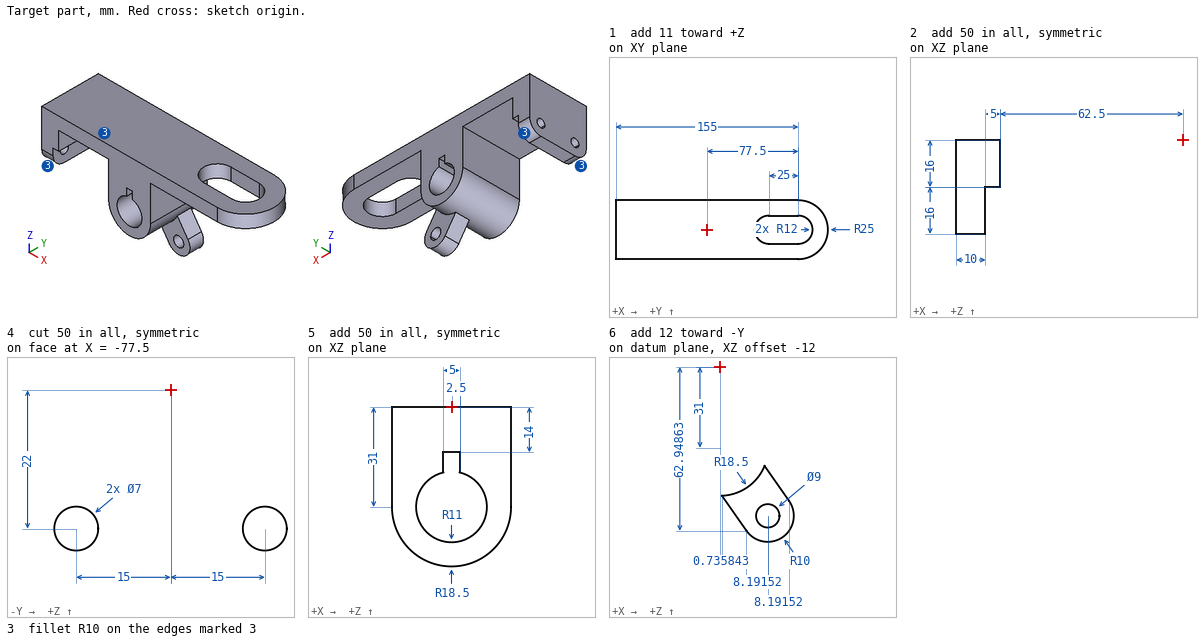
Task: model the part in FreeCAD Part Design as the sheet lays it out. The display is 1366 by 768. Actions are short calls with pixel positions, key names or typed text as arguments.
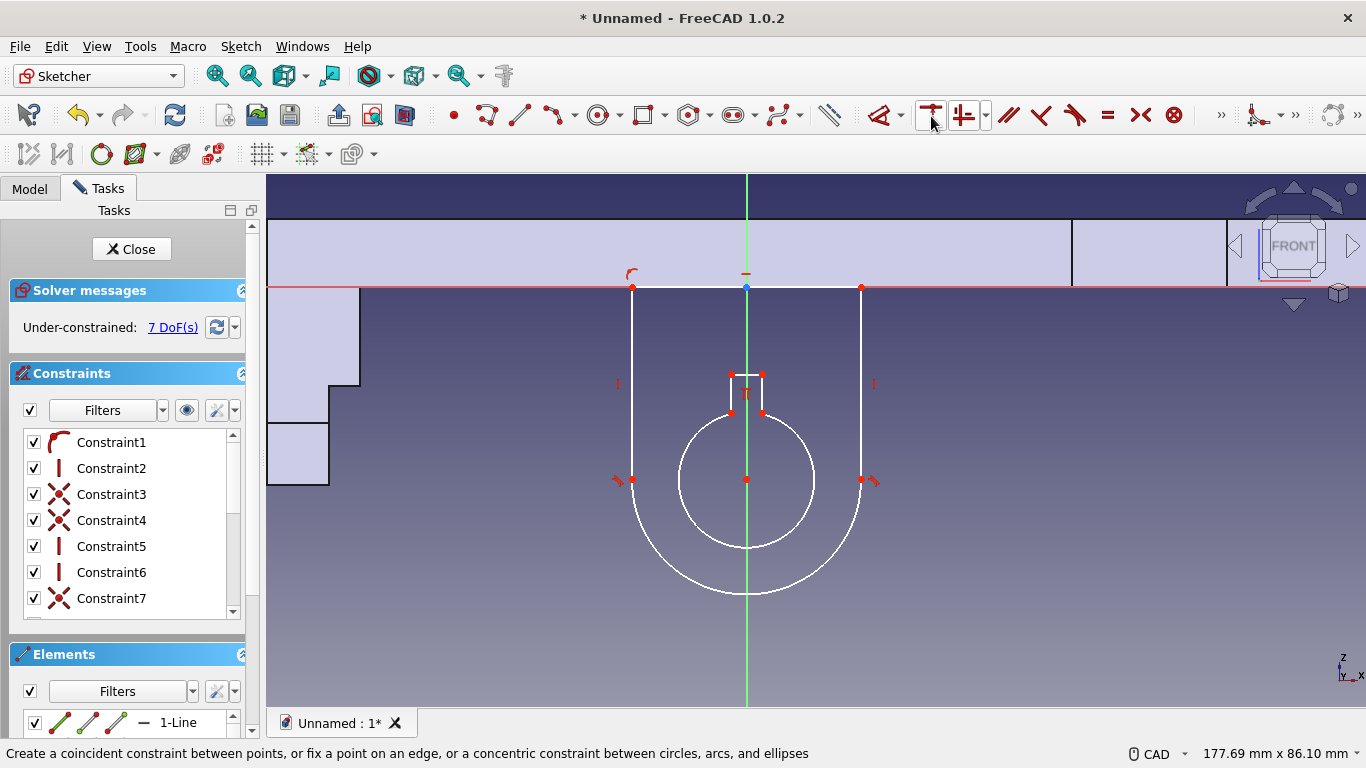
click(747, 480)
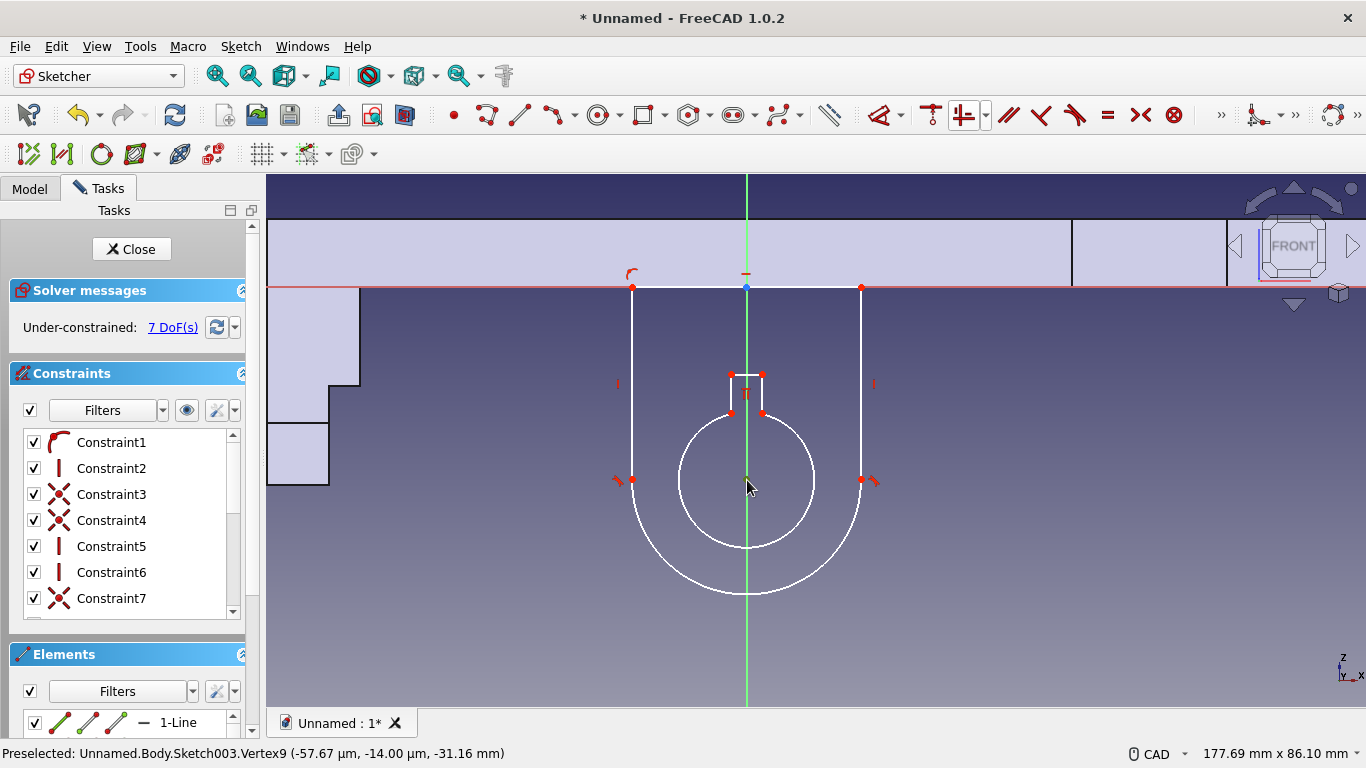
click(747, 645)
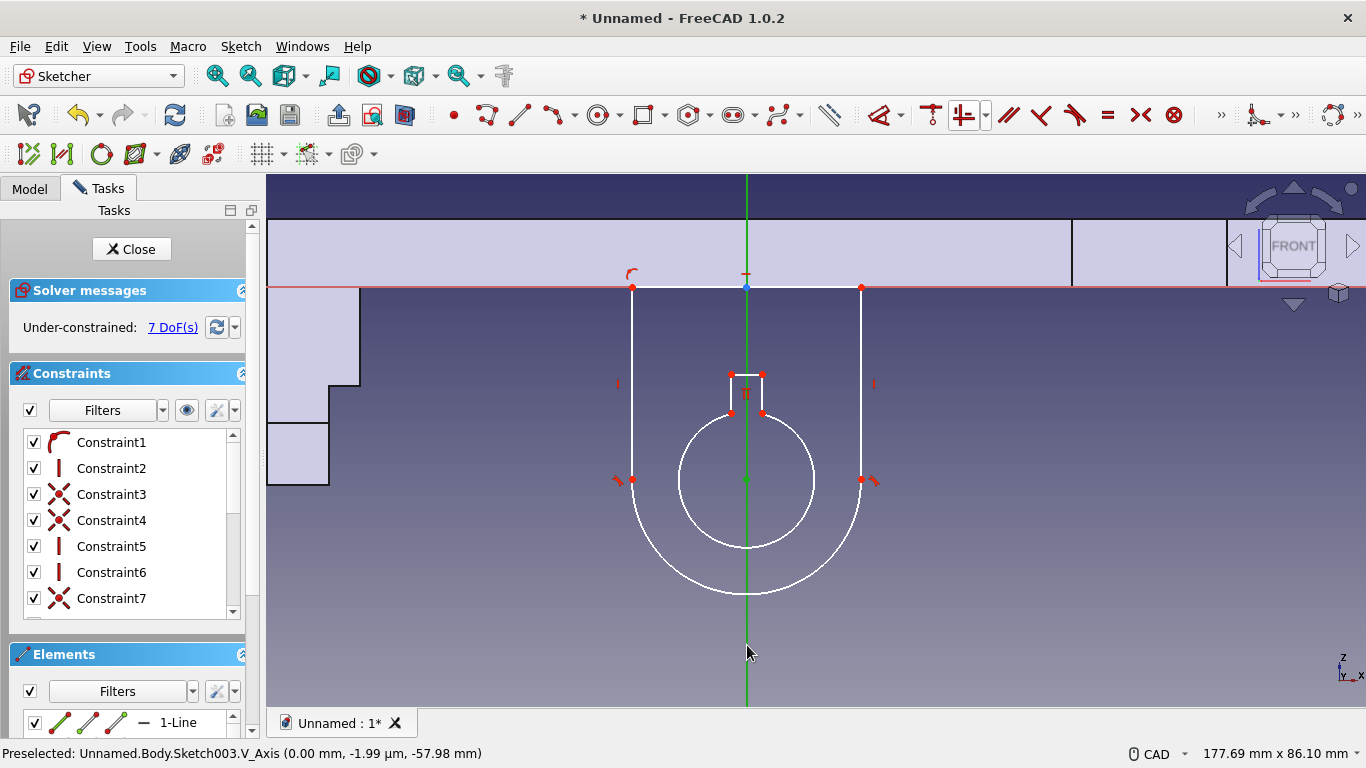
key(c)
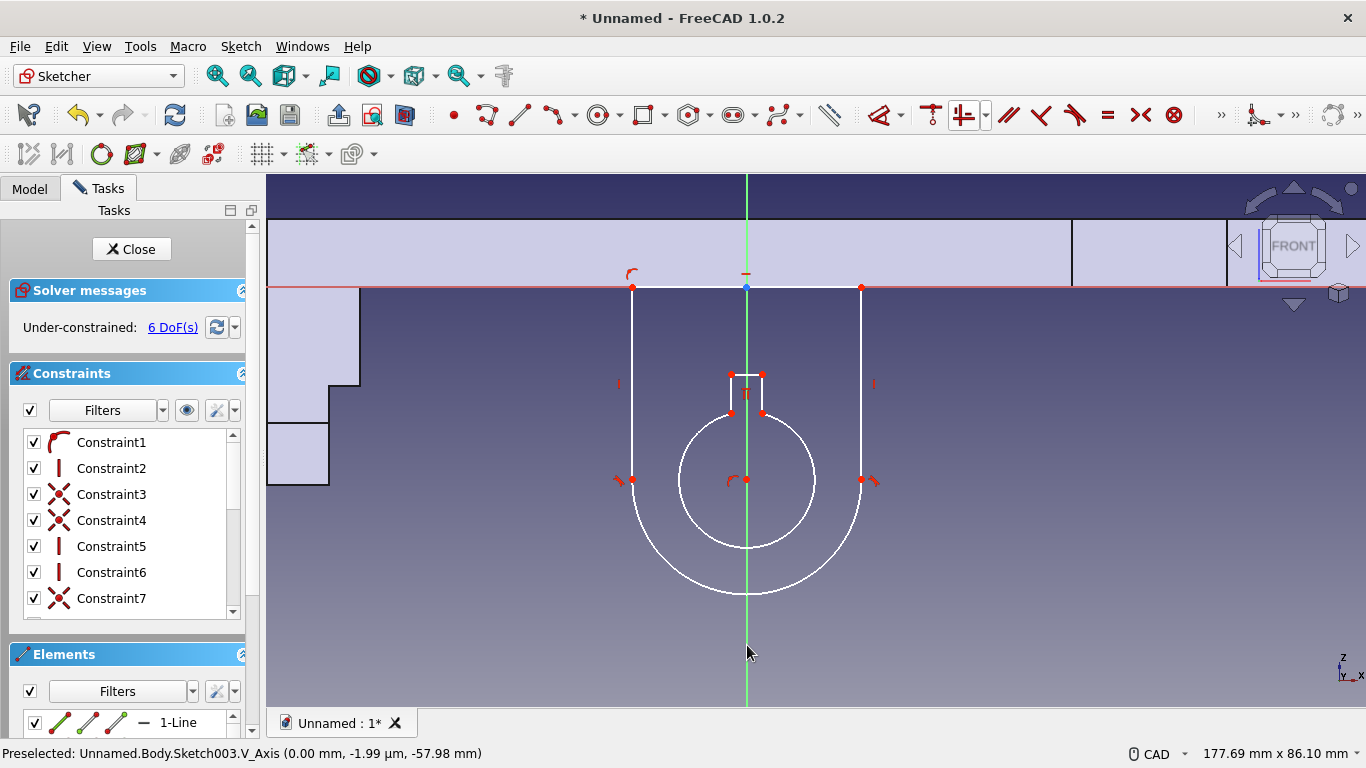
click(878, 116)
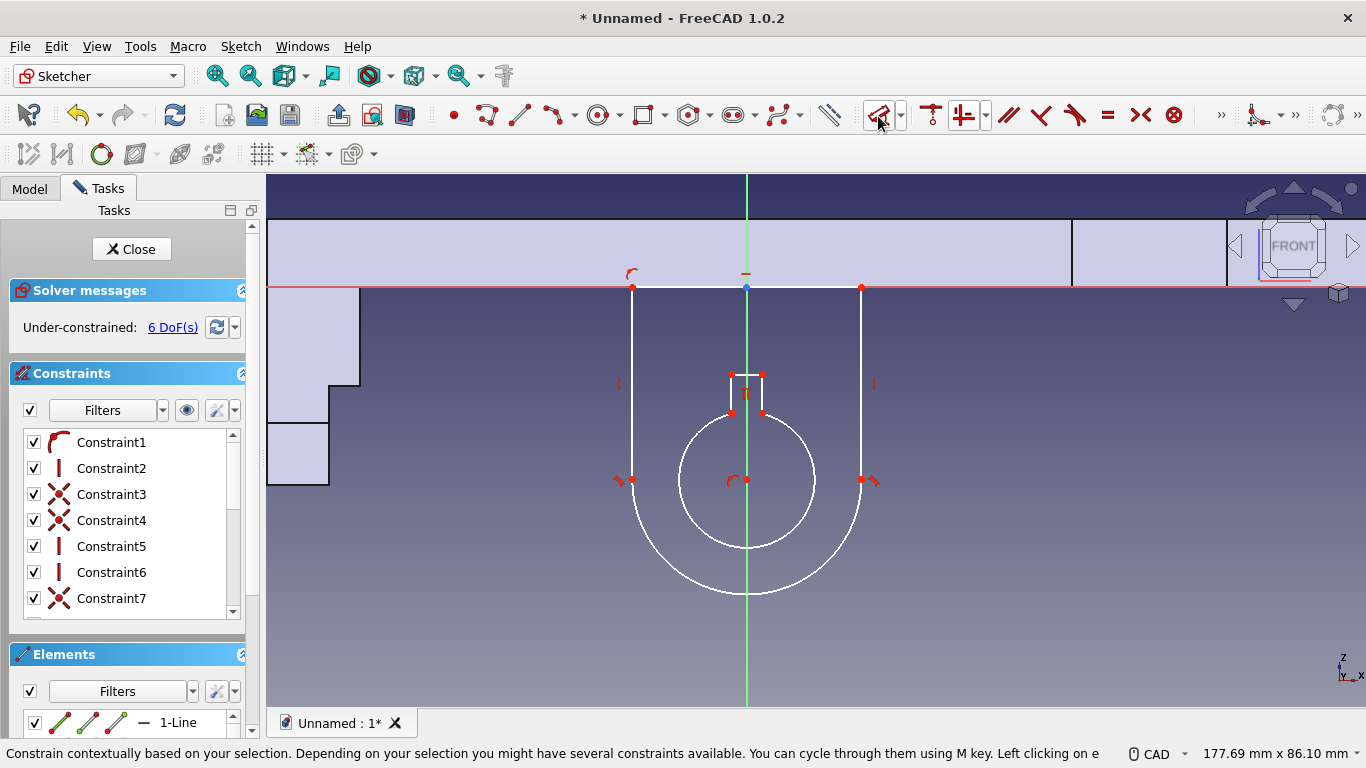
click(680, 573)
click(661, 599)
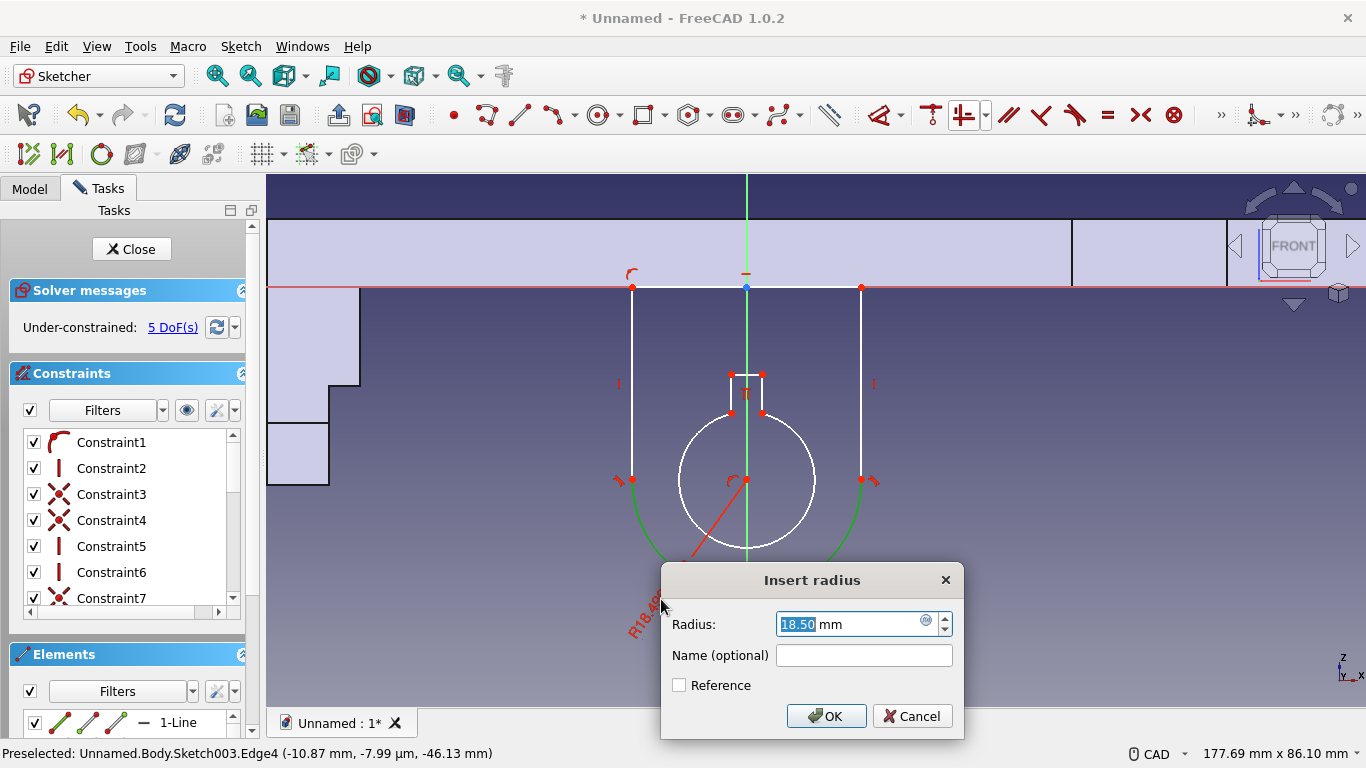
text(18.5)
key(Return)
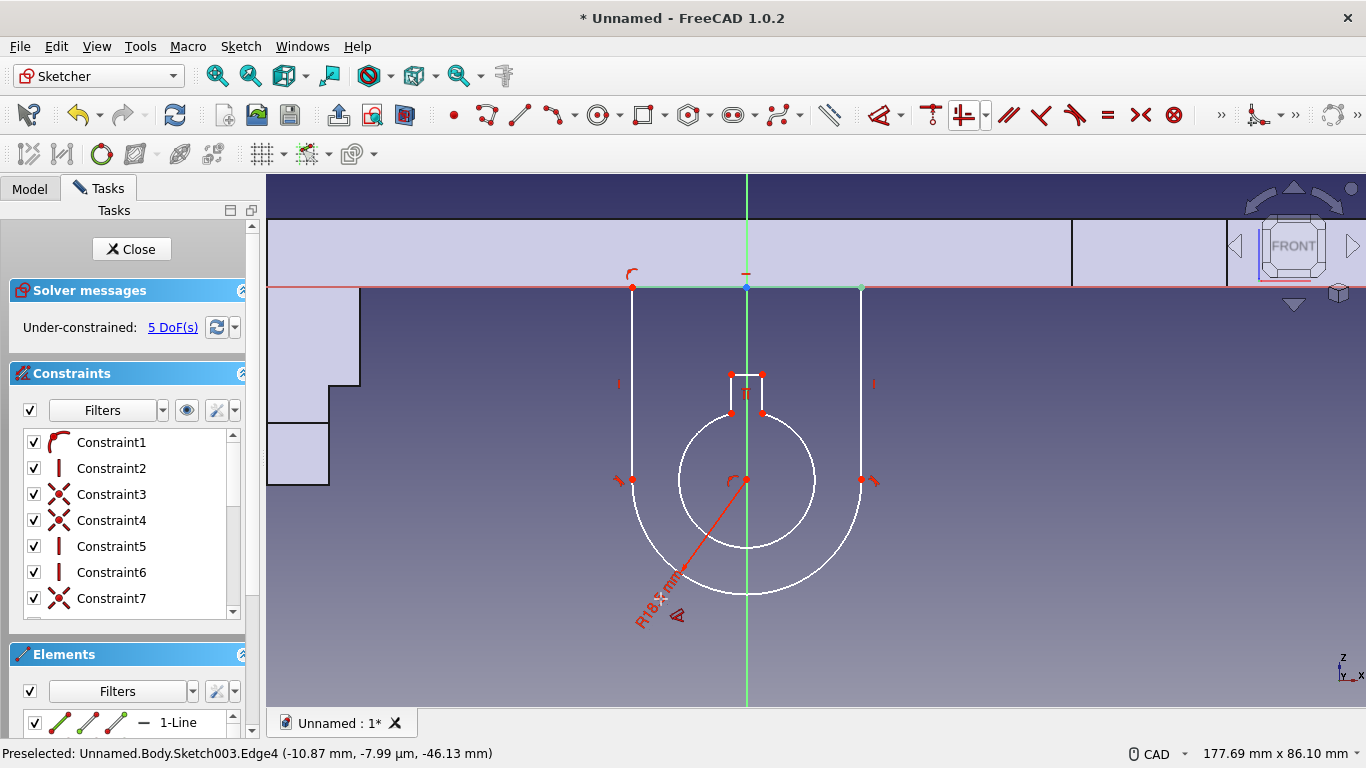
click(685, 507)
click(656, 520)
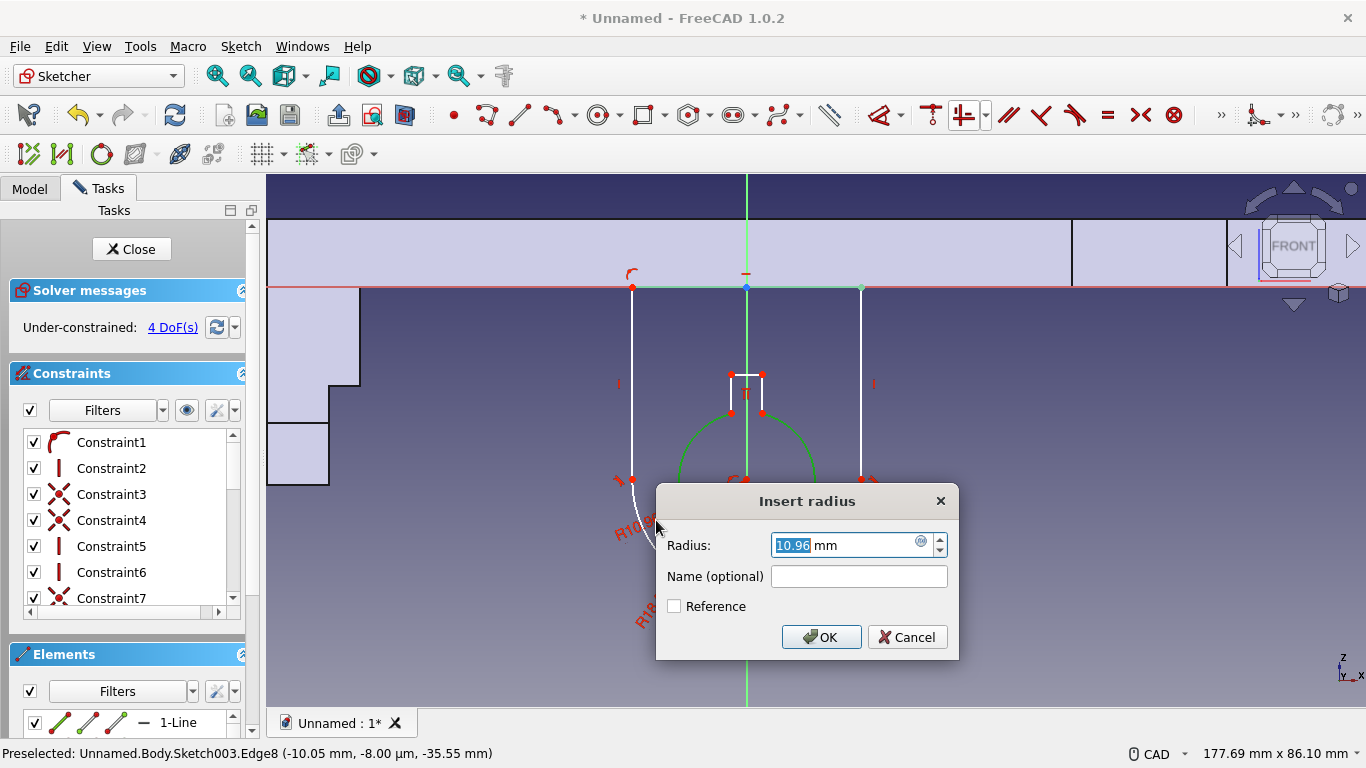
text(11)
key(Return)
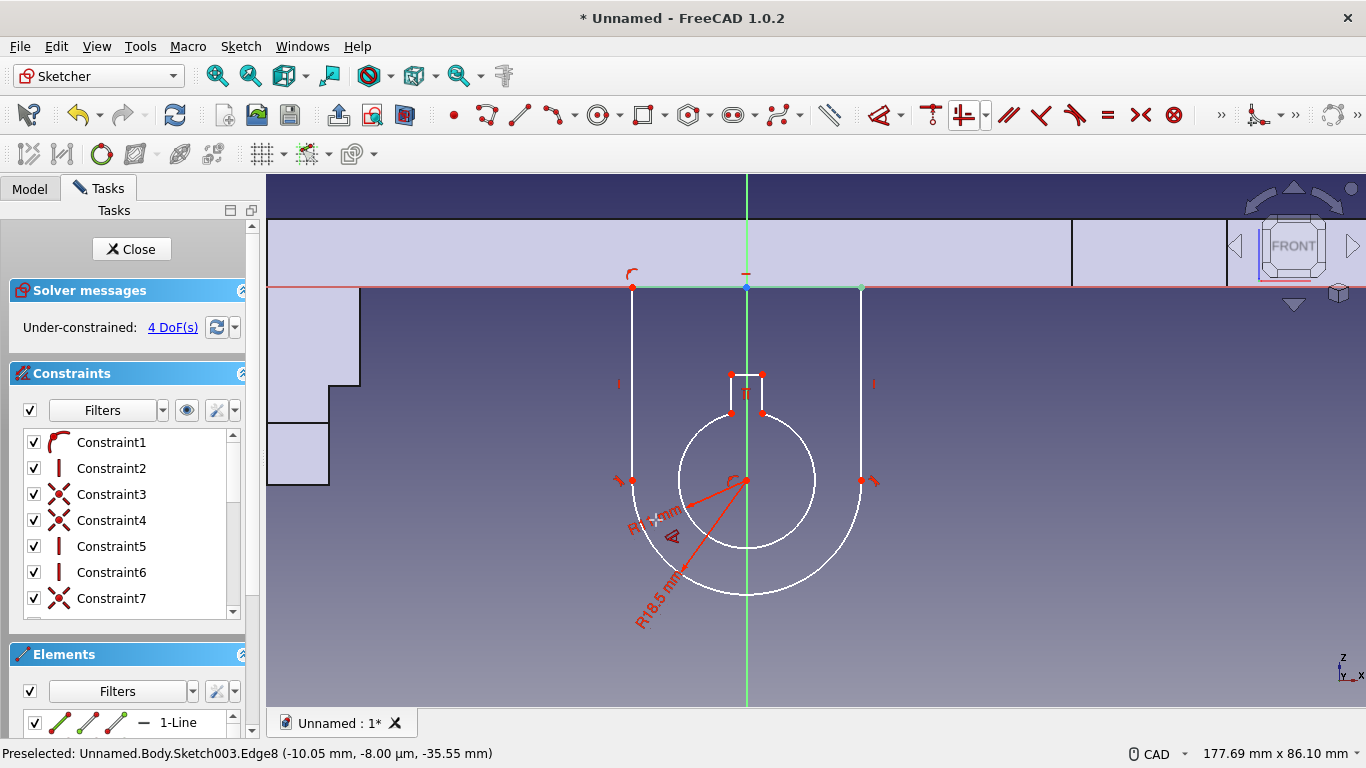
scroll(750, 375, up, 2)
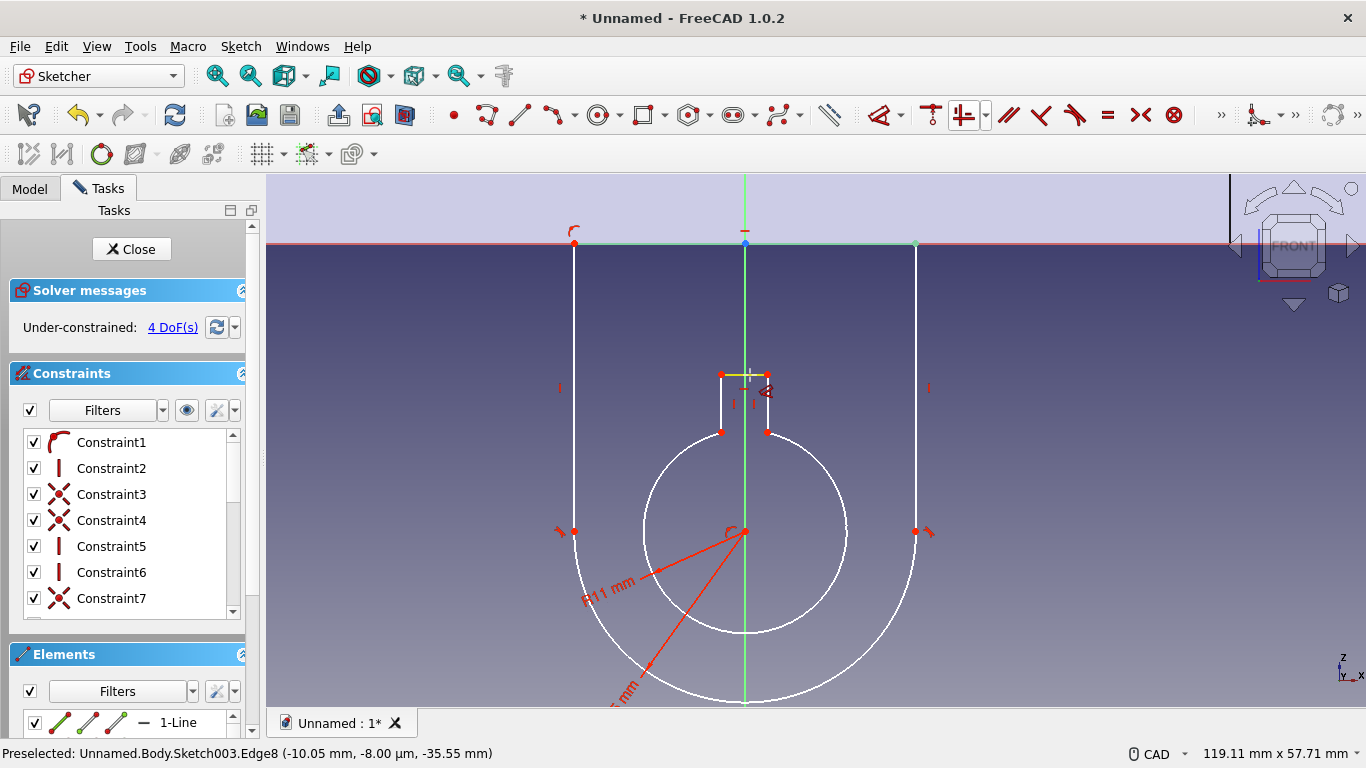
click(749, 375)
click(728, 341)